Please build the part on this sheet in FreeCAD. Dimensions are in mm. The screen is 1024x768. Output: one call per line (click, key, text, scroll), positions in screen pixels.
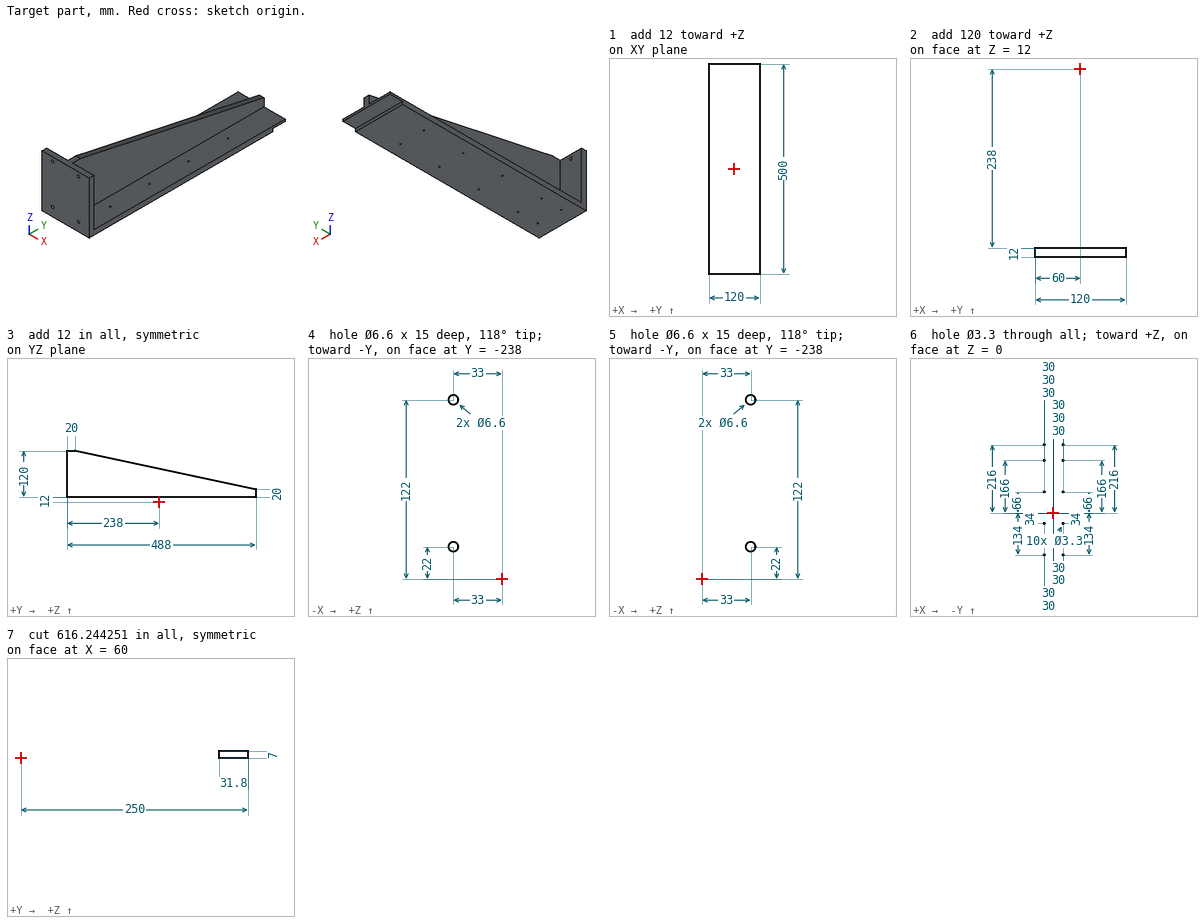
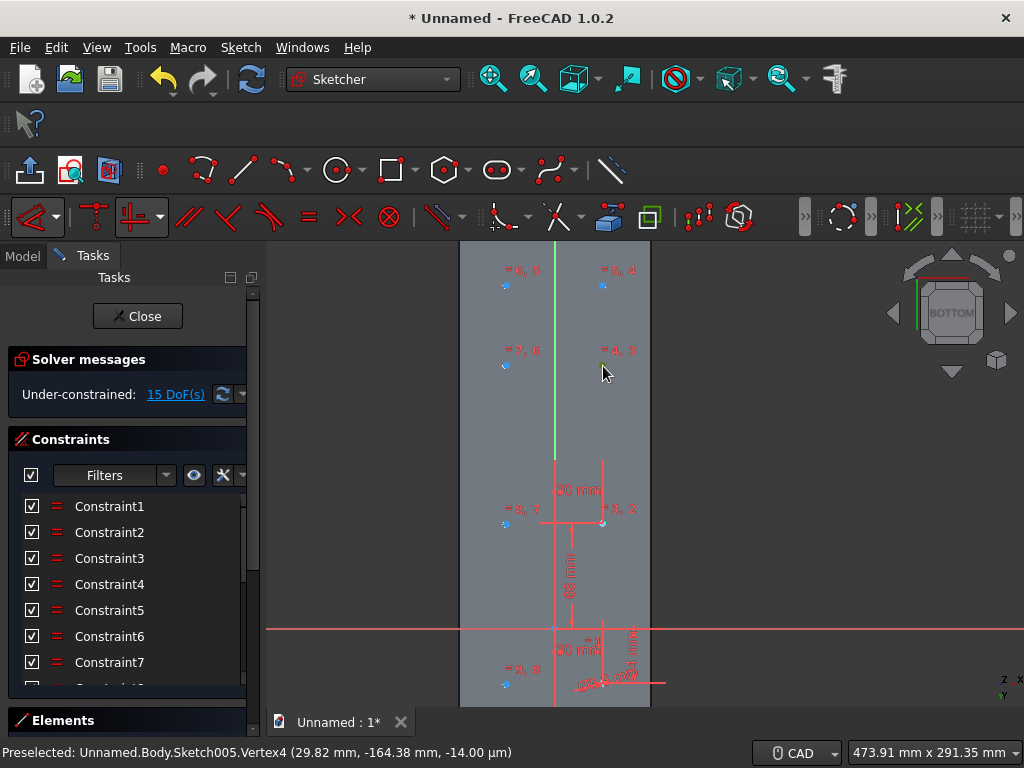
click(58, 218)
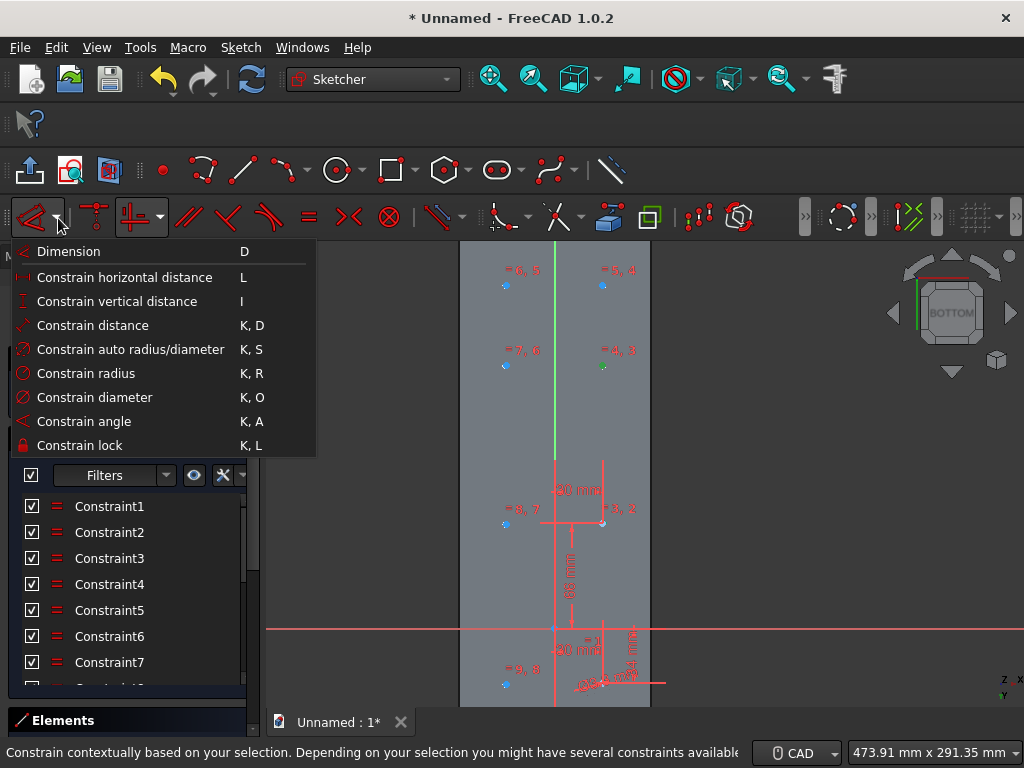
click(164, 277)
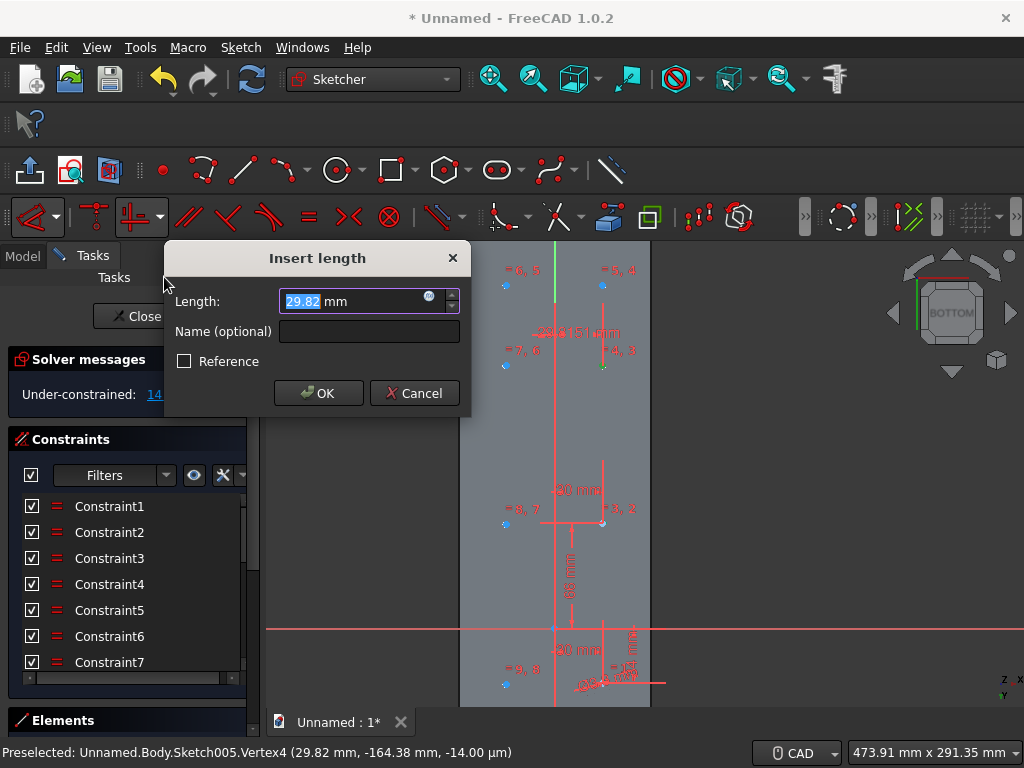
text(30)
key(Return)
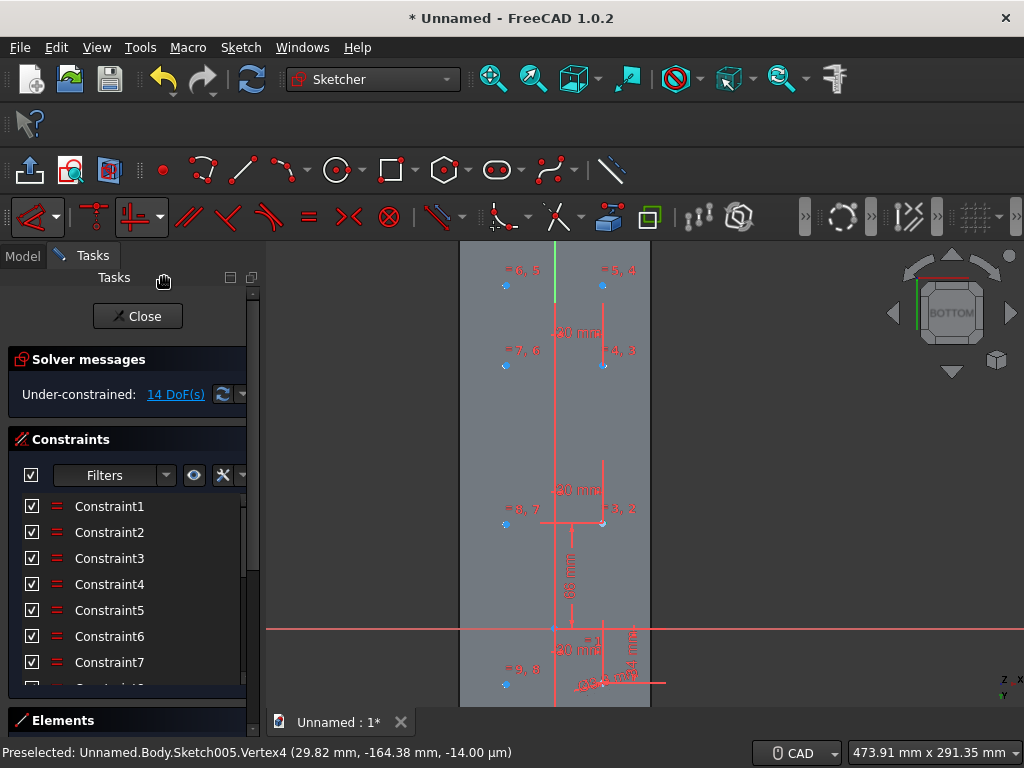
click(603, 286)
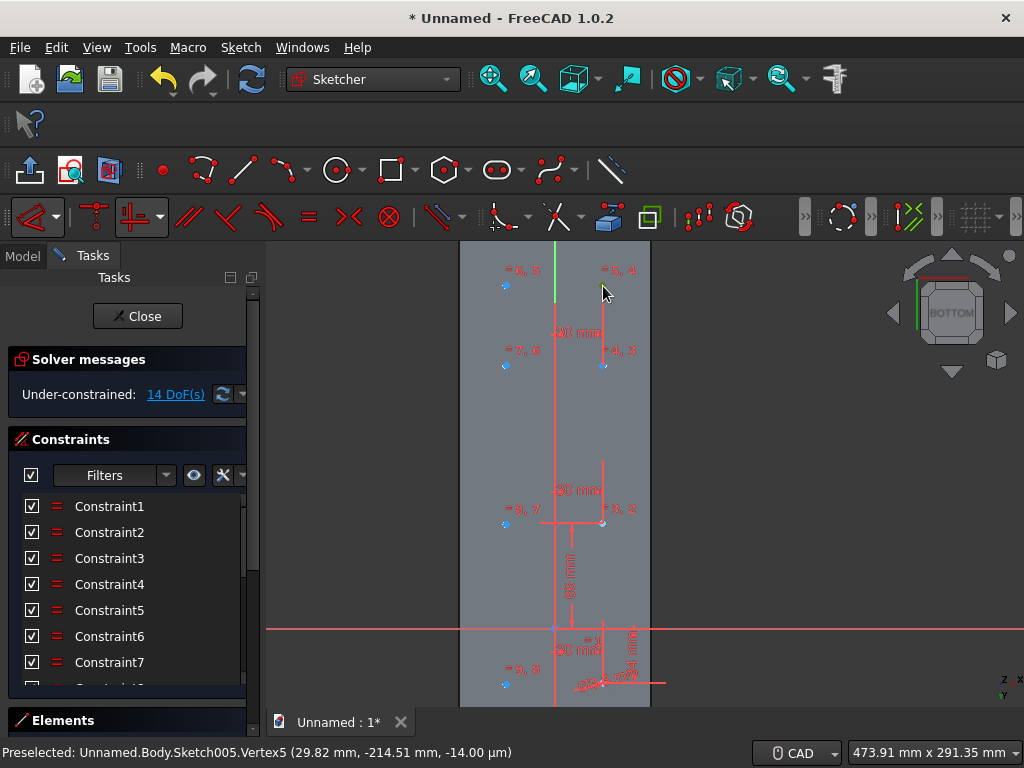
click(58, 218)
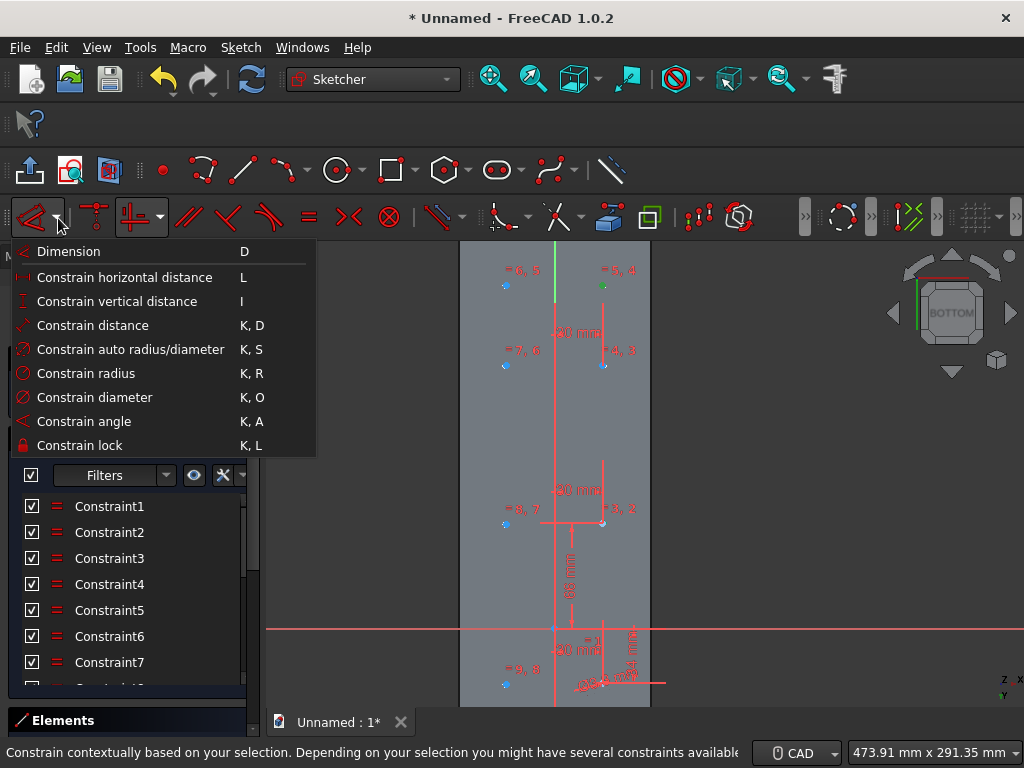
click(164, 277)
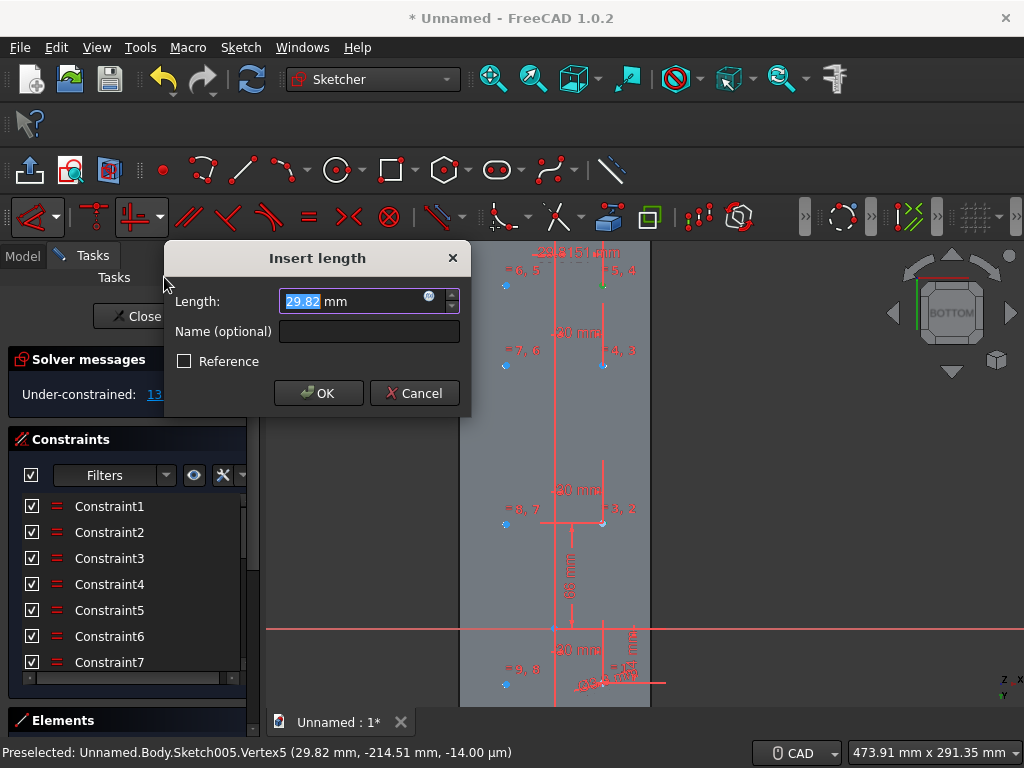
text(30)
key(Return)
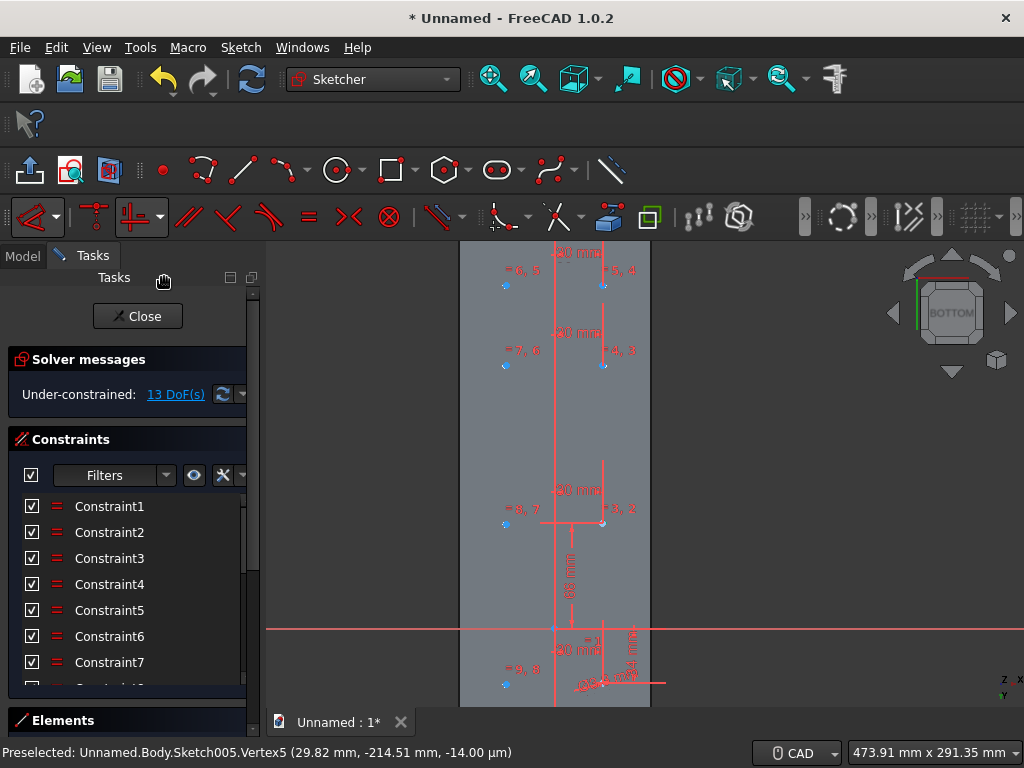
click(506, 286)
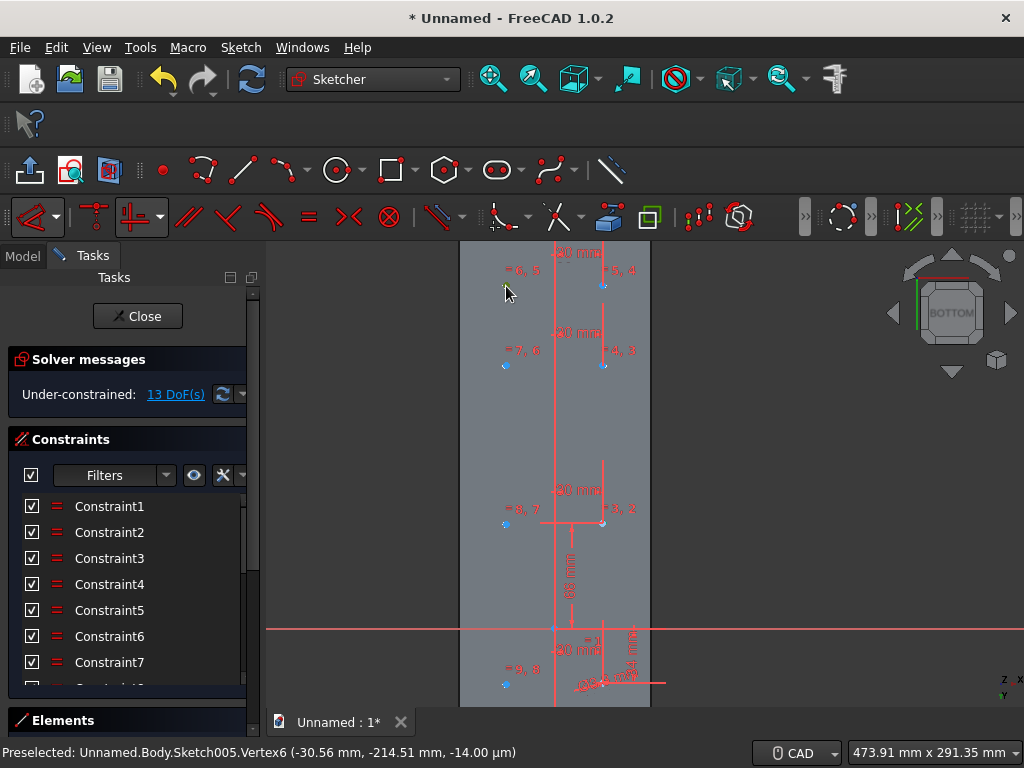
click(58, 218)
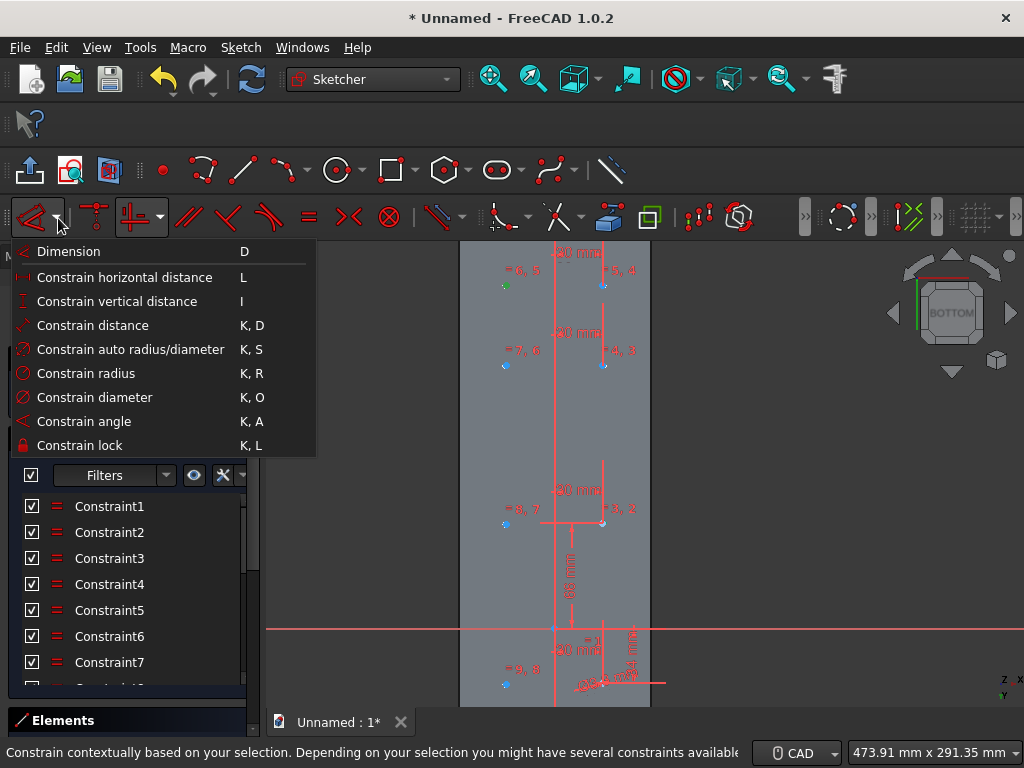
click(164, 277)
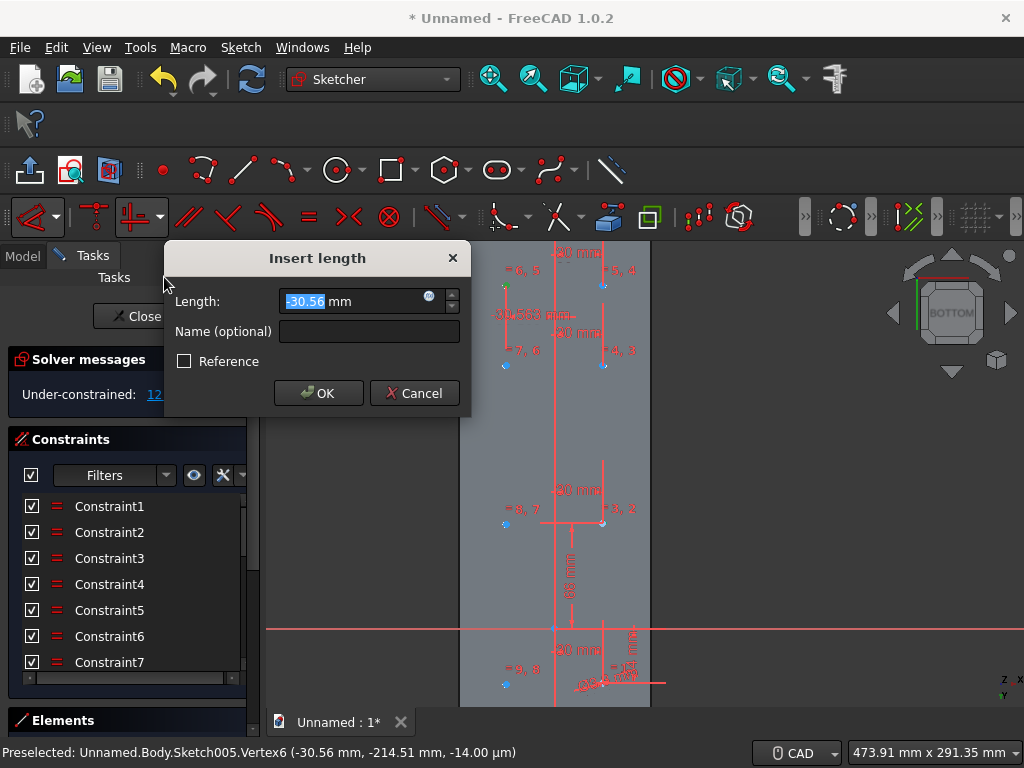
text(-30)
key(Return)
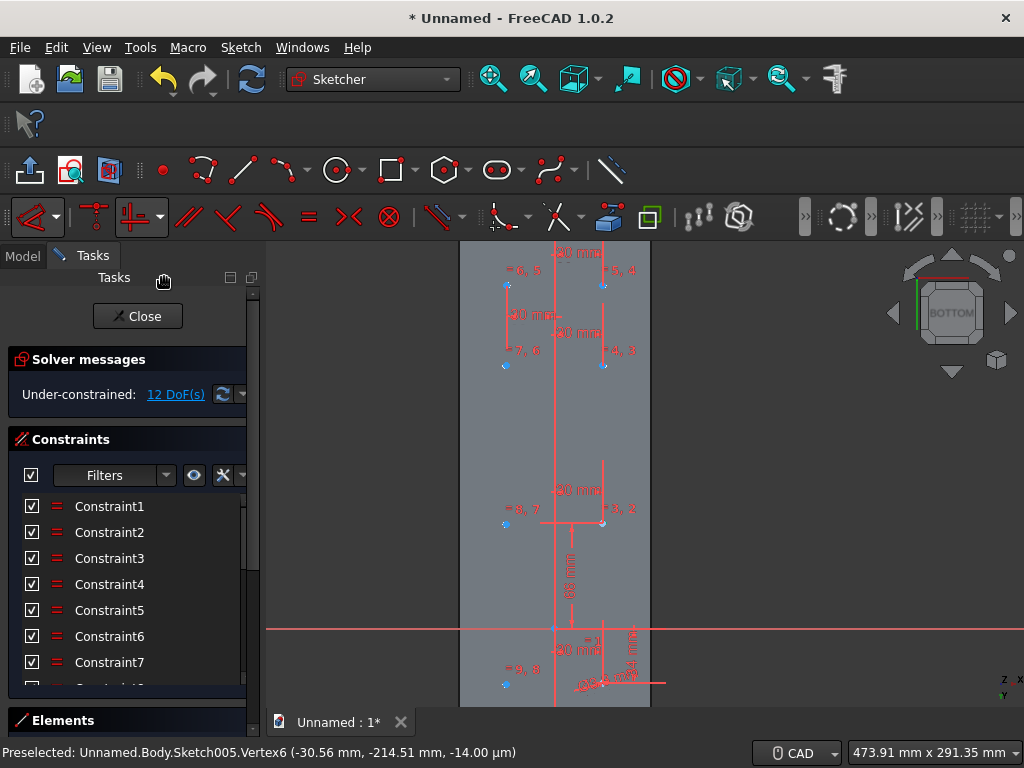
click(506, 366)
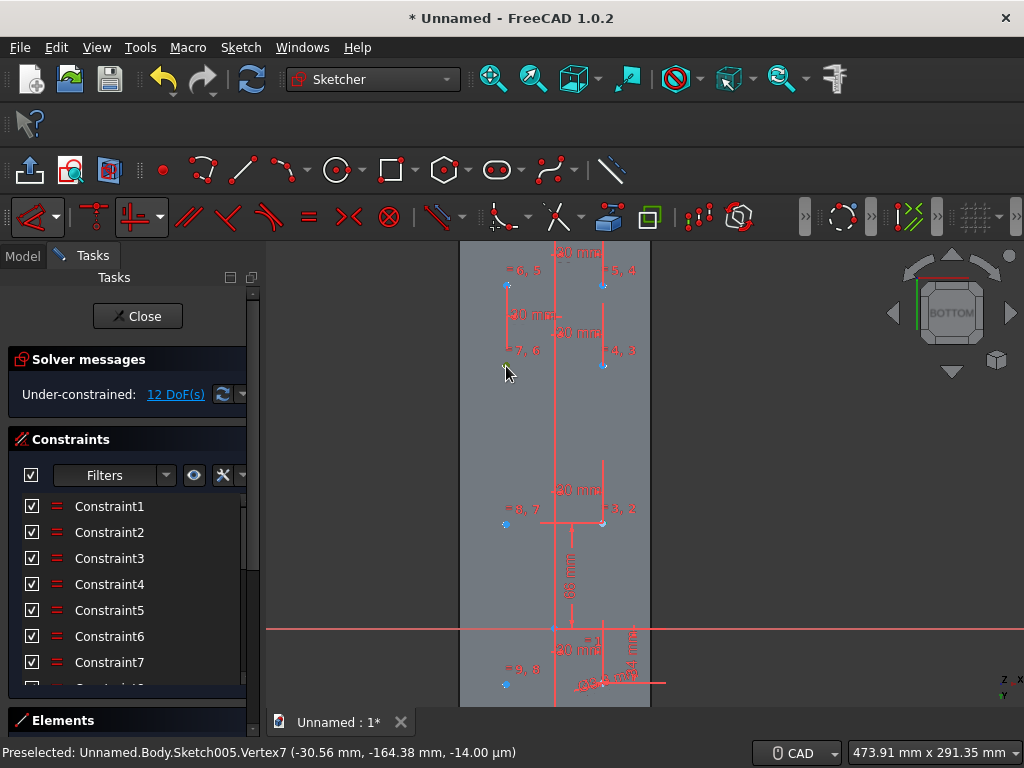
key(l)